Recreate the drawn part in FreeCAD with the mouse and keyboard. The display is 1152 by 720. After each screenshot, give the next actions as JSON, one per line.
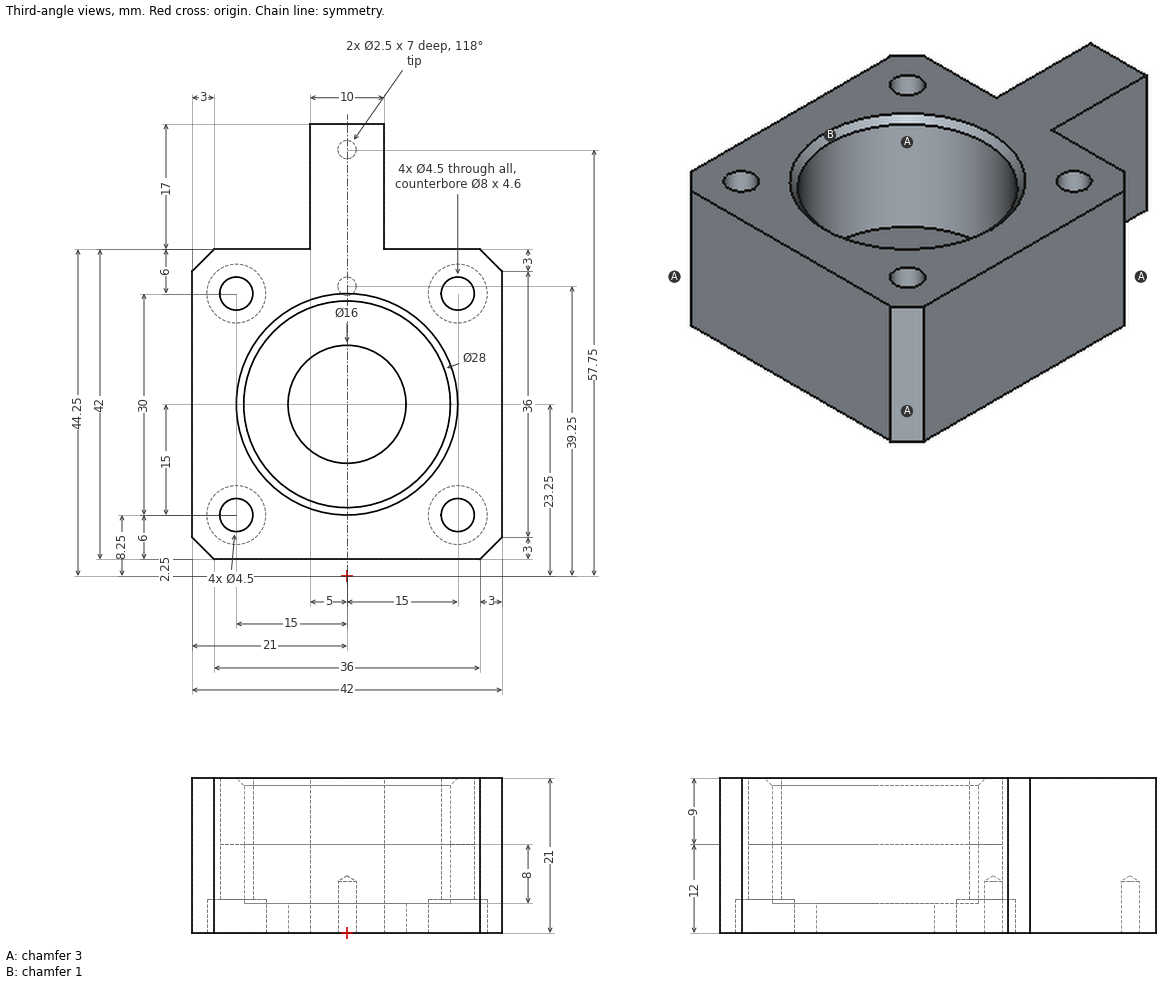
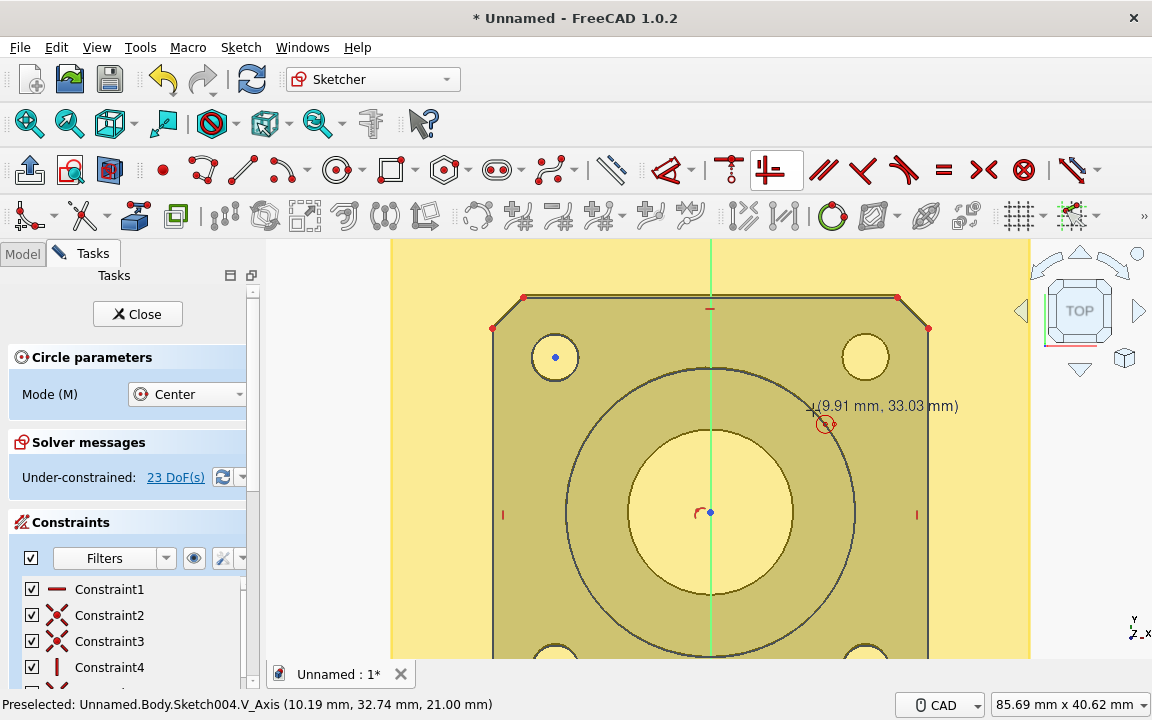
{"action": "left_click", "coordinate": [866, 357]}
{"action": "left_click", "coordinate": [882, 341]}
{"action": "key", "text": "Escape"}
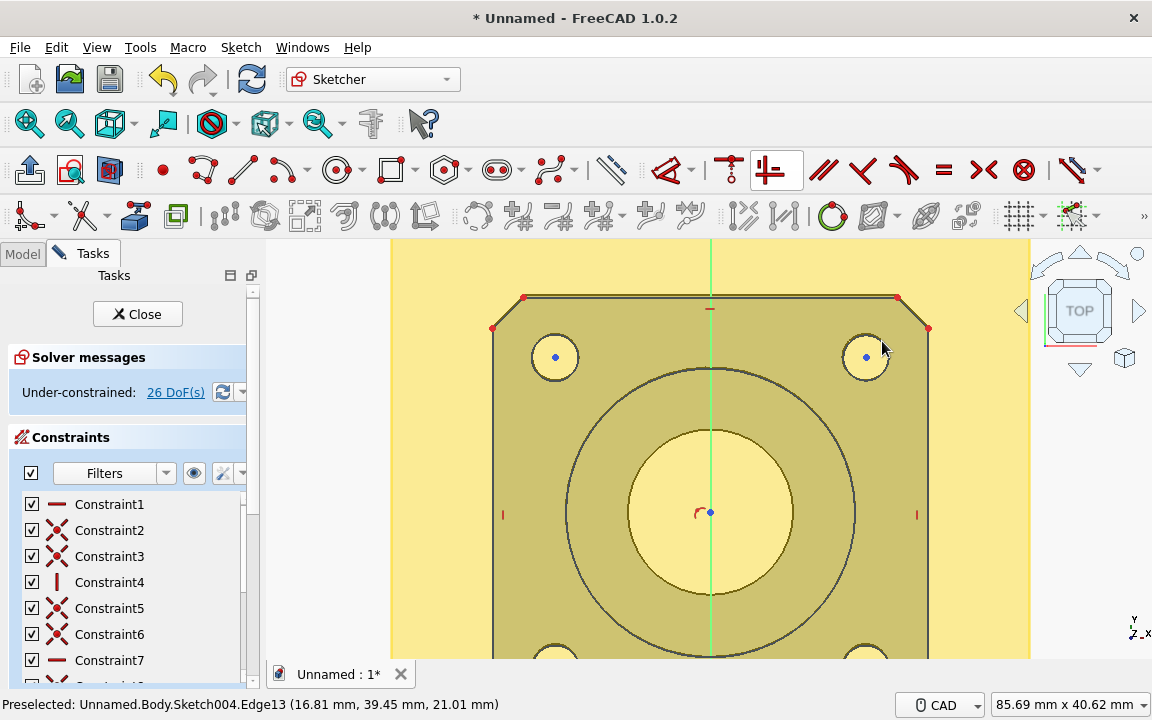
{"action": "scroll", "coordinate": [555, 358], "scroll_direction": "down", "scroll_amount": 3}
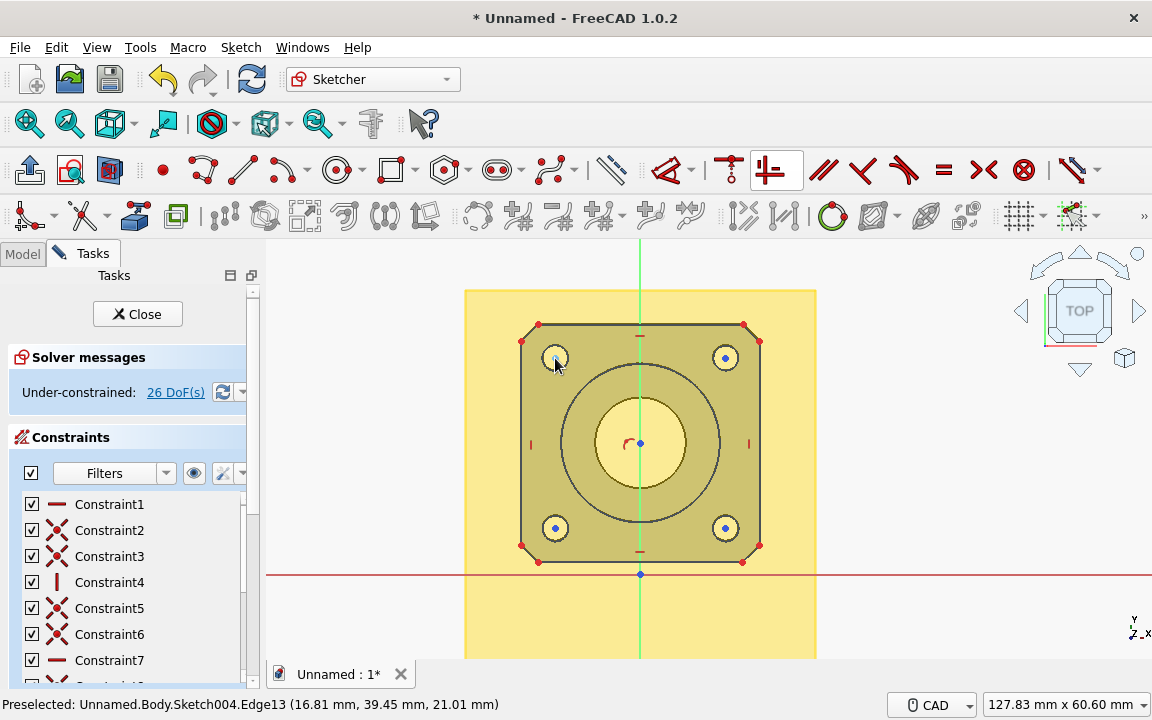
{"action": "left_click", "coordinate": [565, 520]}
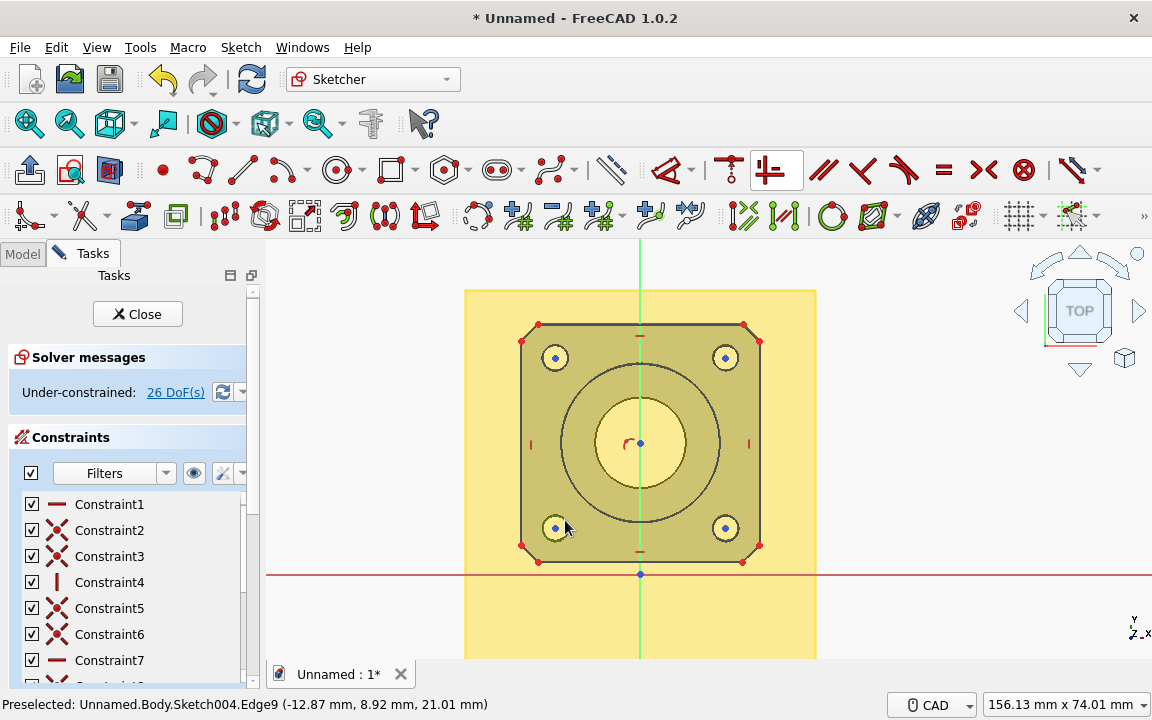
{"action": "left_click", "coordinate": [735, 520]}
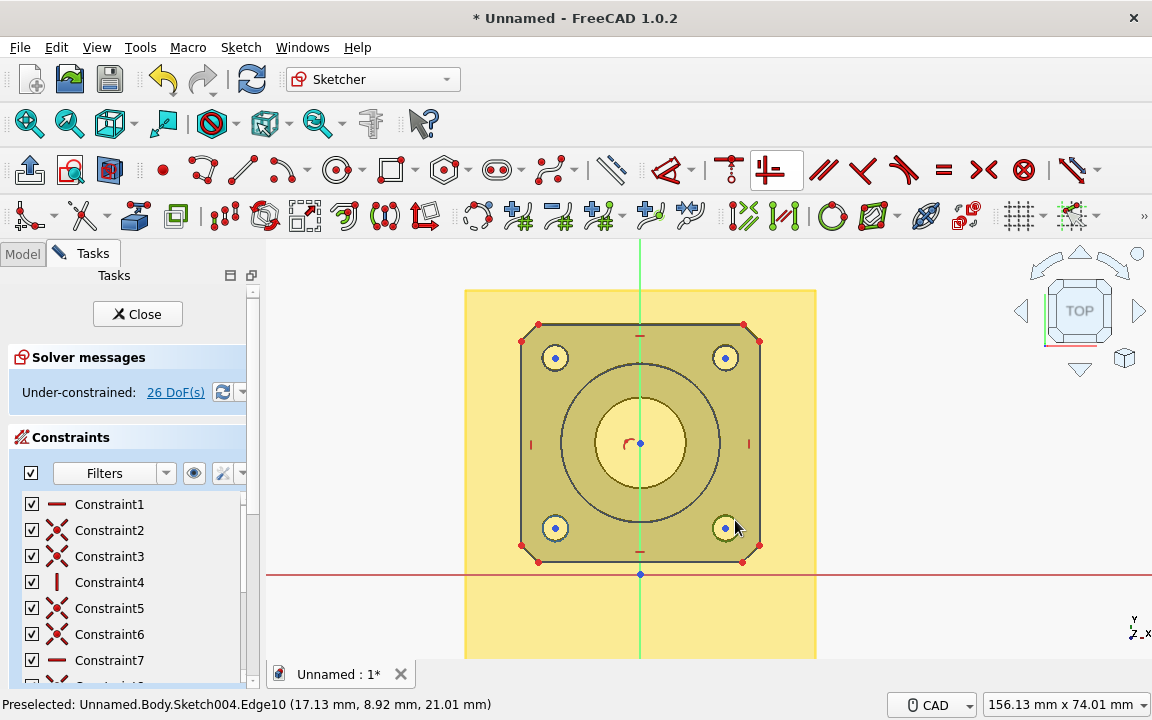
{"action": "left_click", "coordinate": [564, 349]}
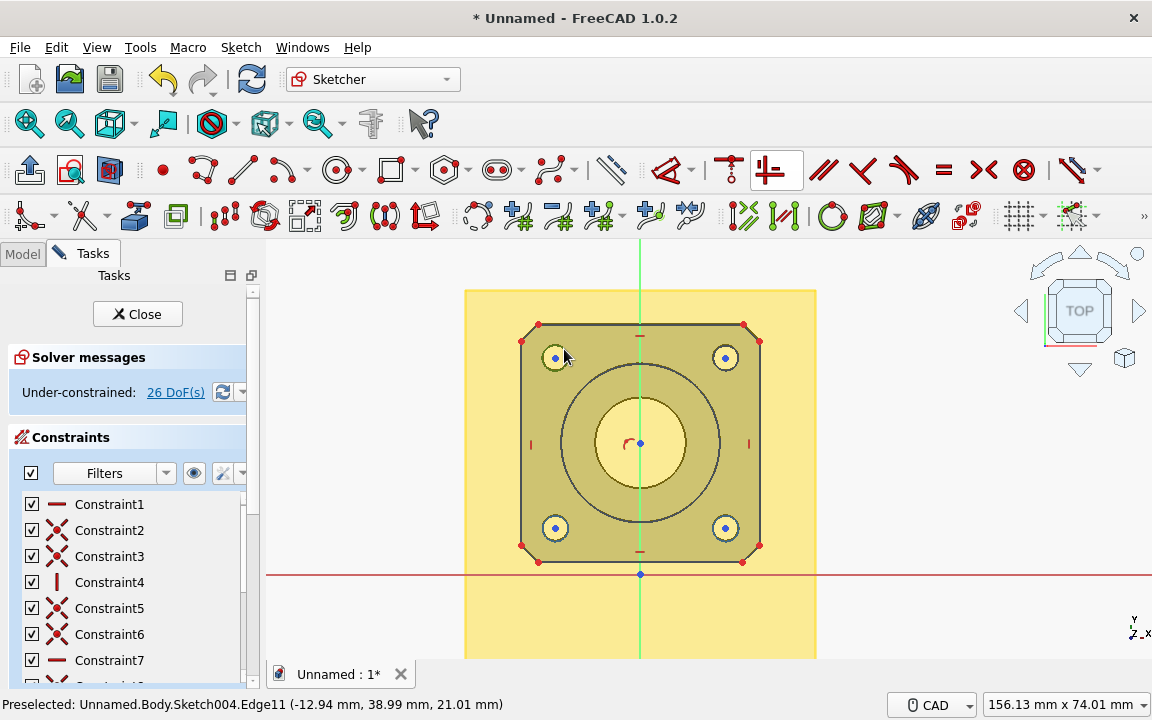
{"action": "left_click", "coordinate": [735, 349]}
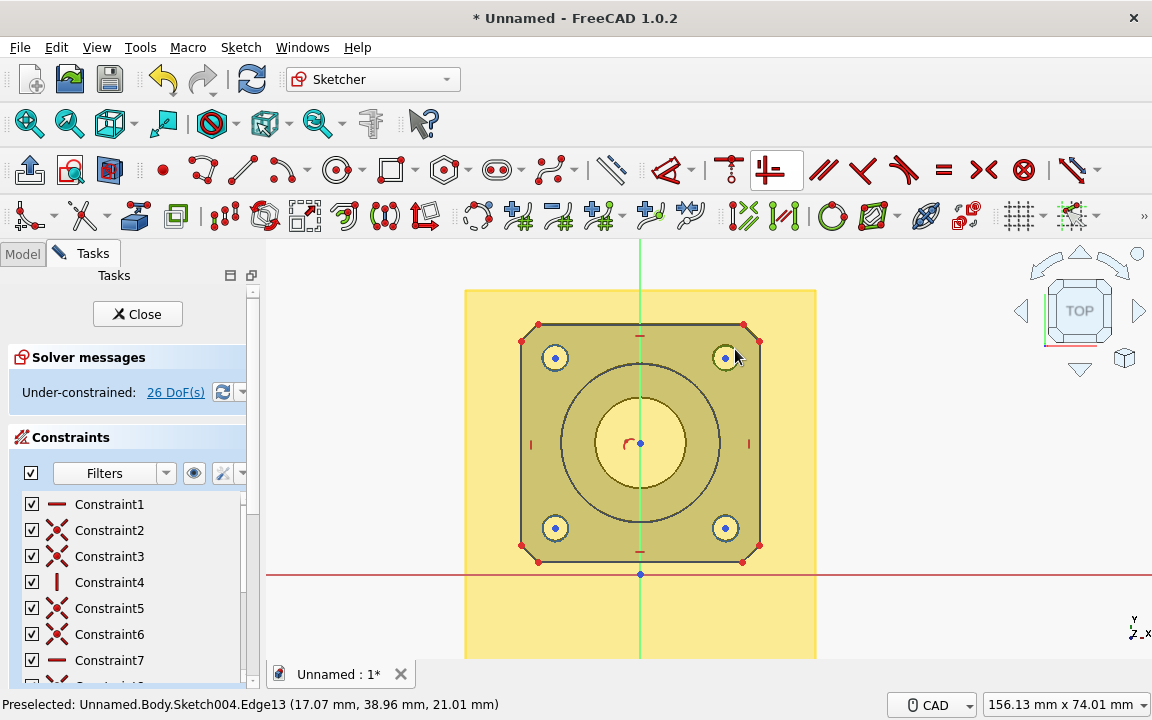
{"action": "left_click", "coordinate": [944, 170]}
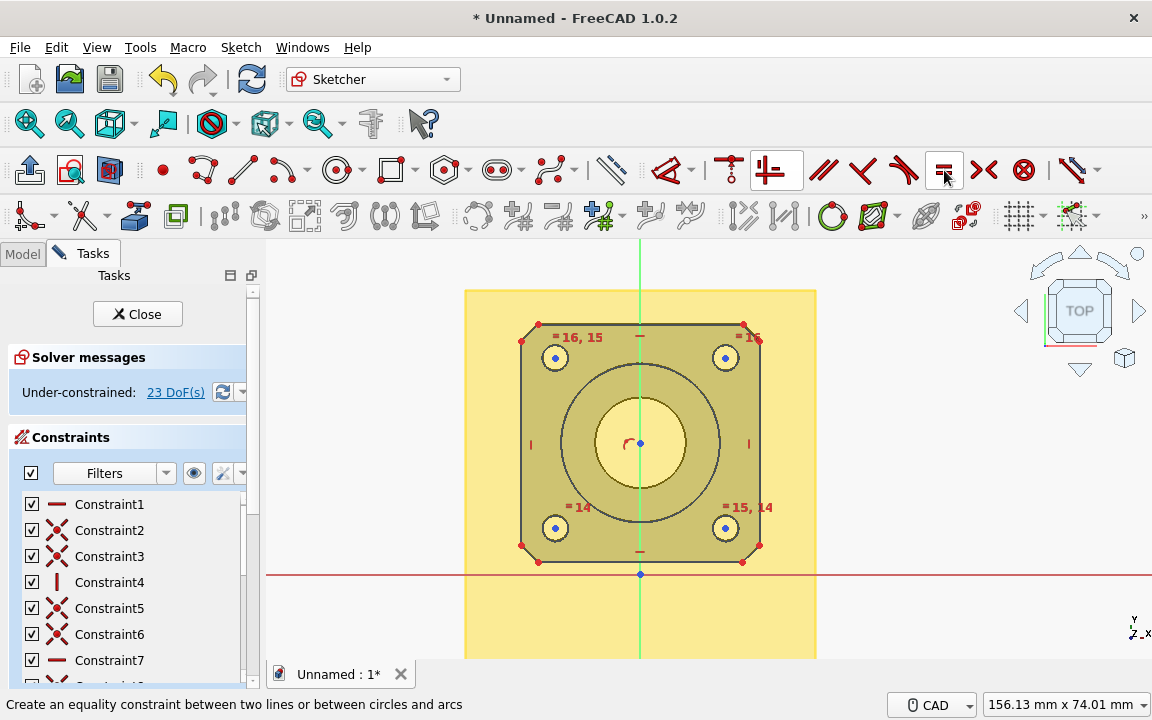
{"action": "left_click", "coordinate": [556, 529]}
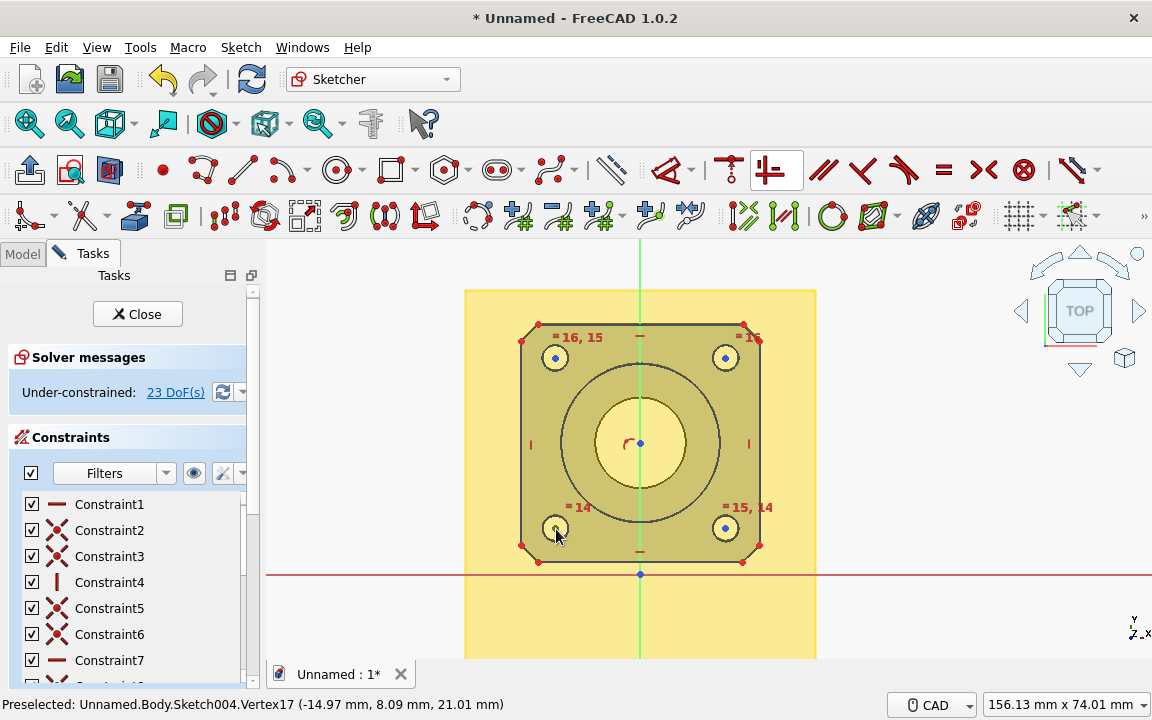
{"action": "left_click", "coordinate": [726, 529]}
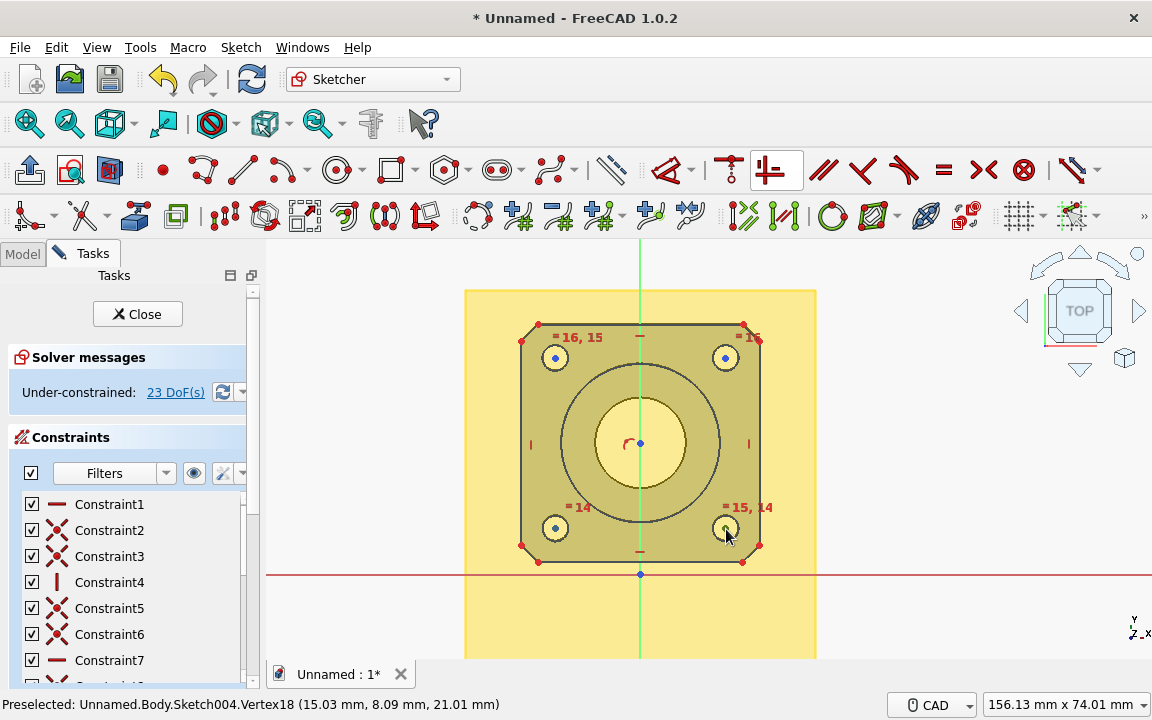
{"action": "left_click", "coordinate": [798, 170]}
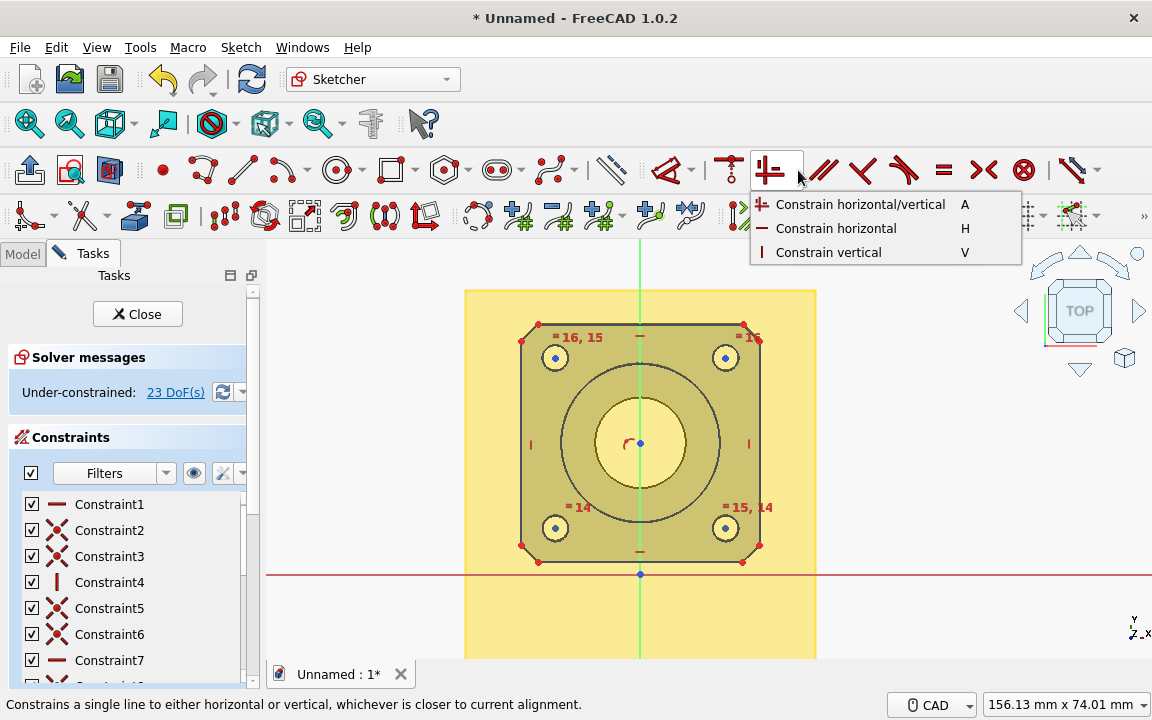
{"action": "left_click", "coordinate": [886, 228]}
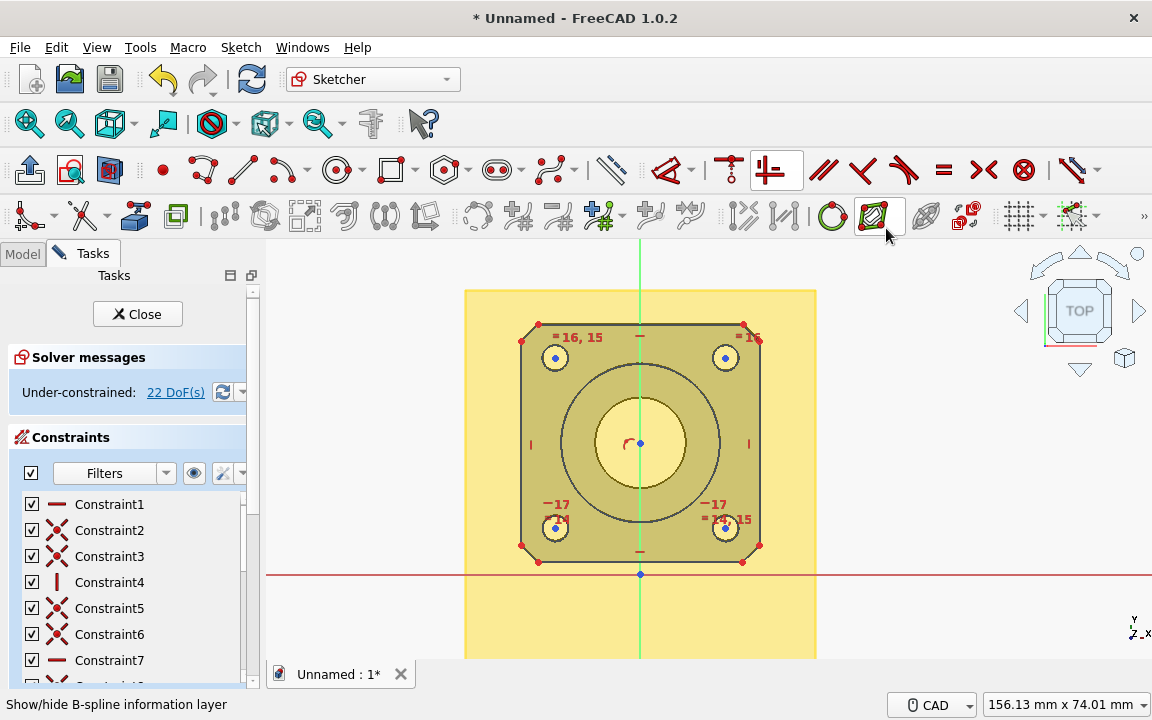
{"action": "left_click", "coordinate": [556, 529]}